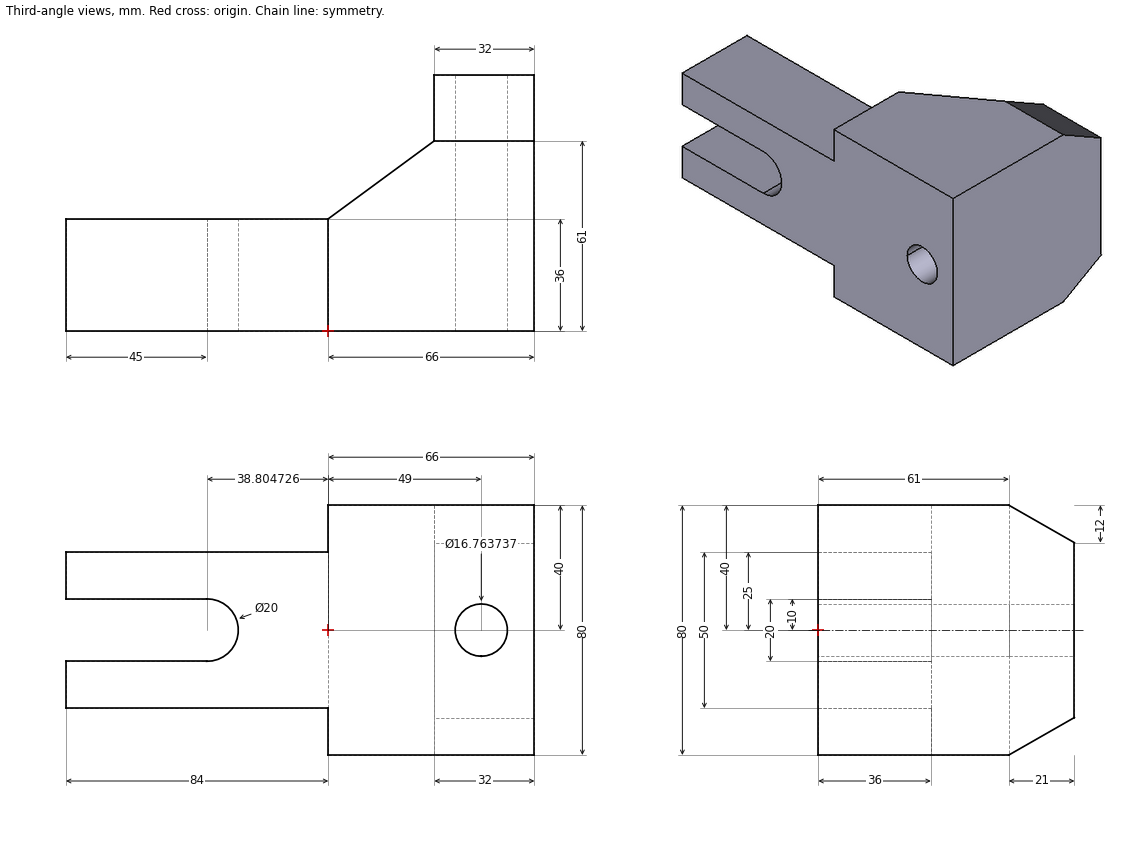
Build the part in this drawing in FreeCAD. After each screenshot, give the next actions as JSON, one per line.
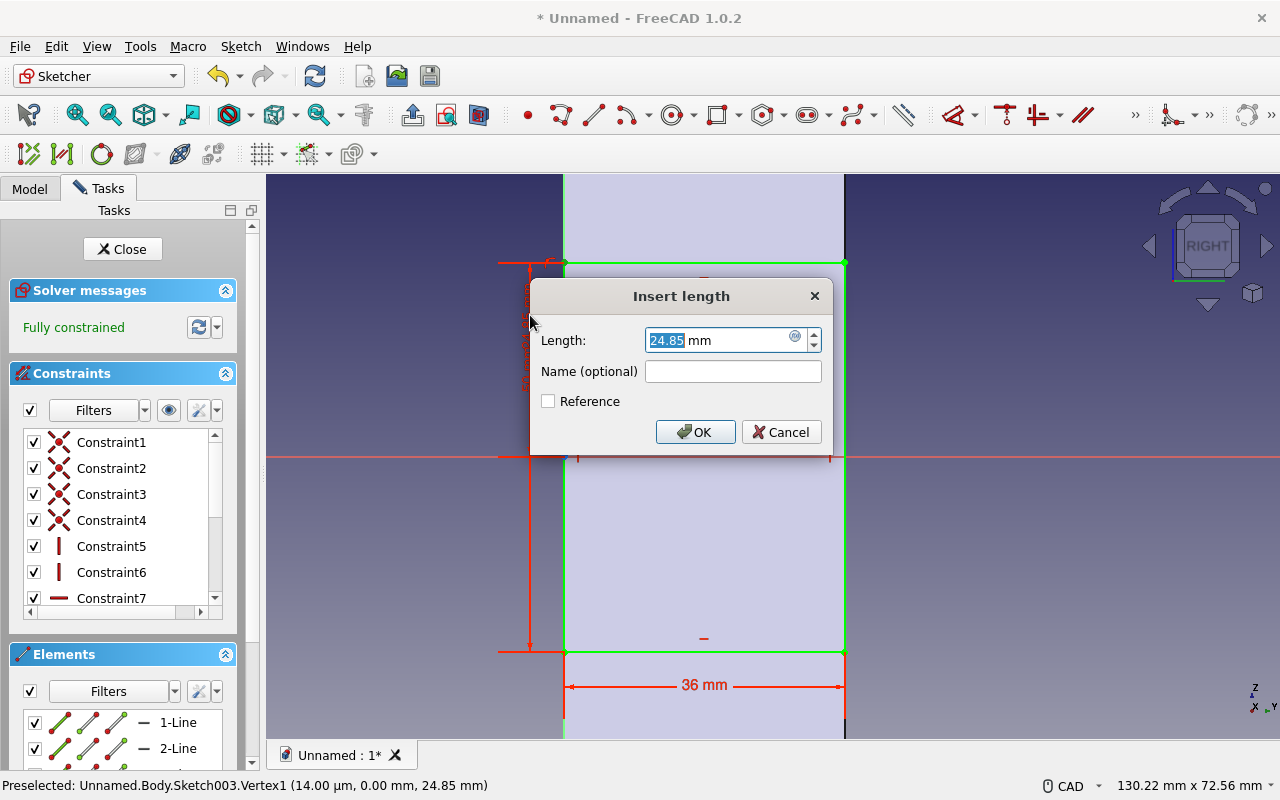
{"action": "type", "text": "25"}
{"action": "key", "text": "Return"}
{"action": "key", "text": "Escape"}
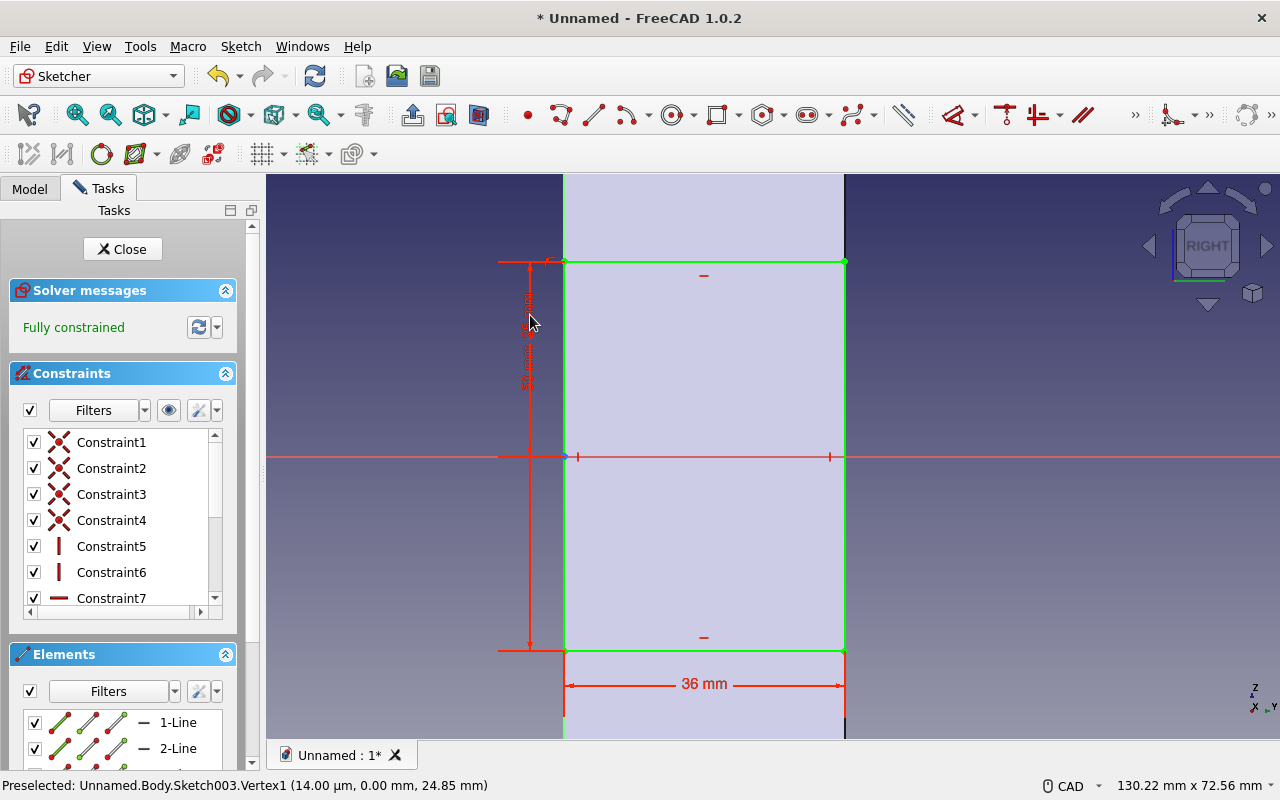
{"action": "left_click", "coordinate": [123, 249]}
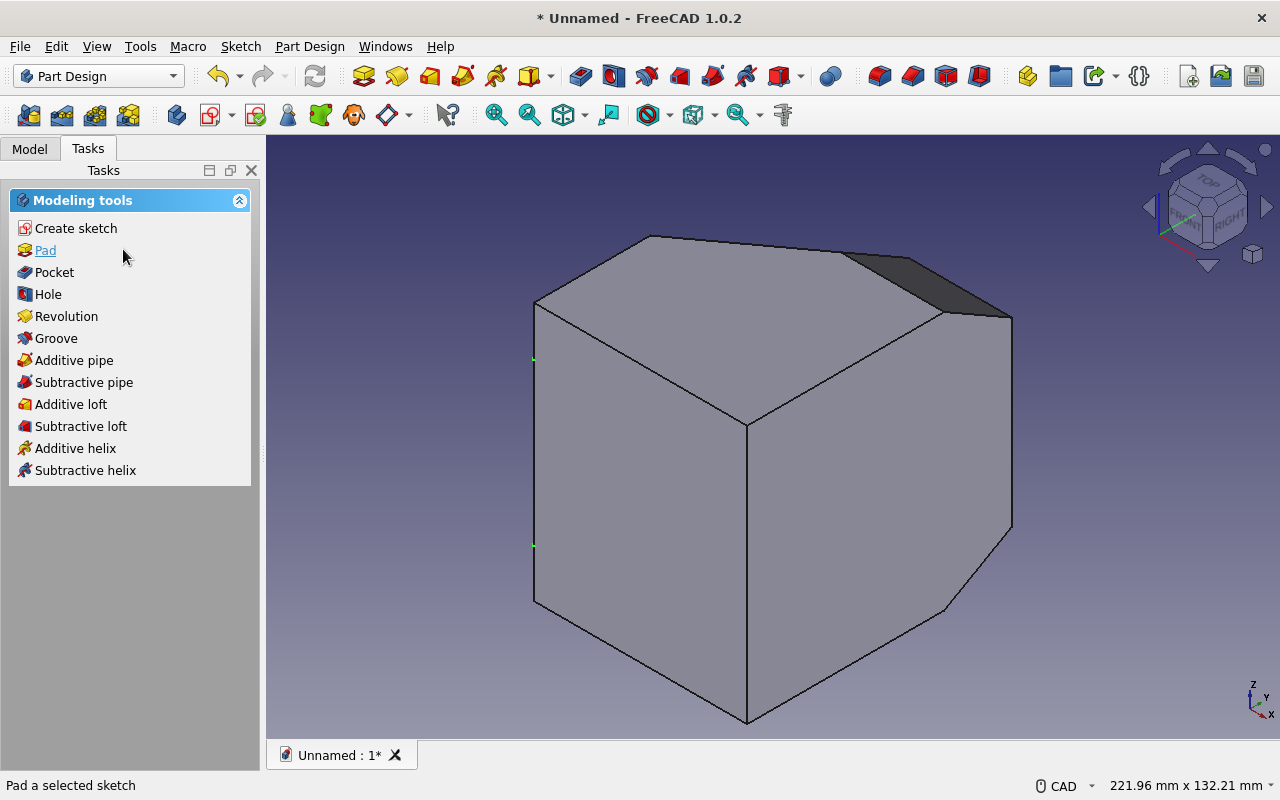
{"action": "left_click", "coordinate": [364, 76]}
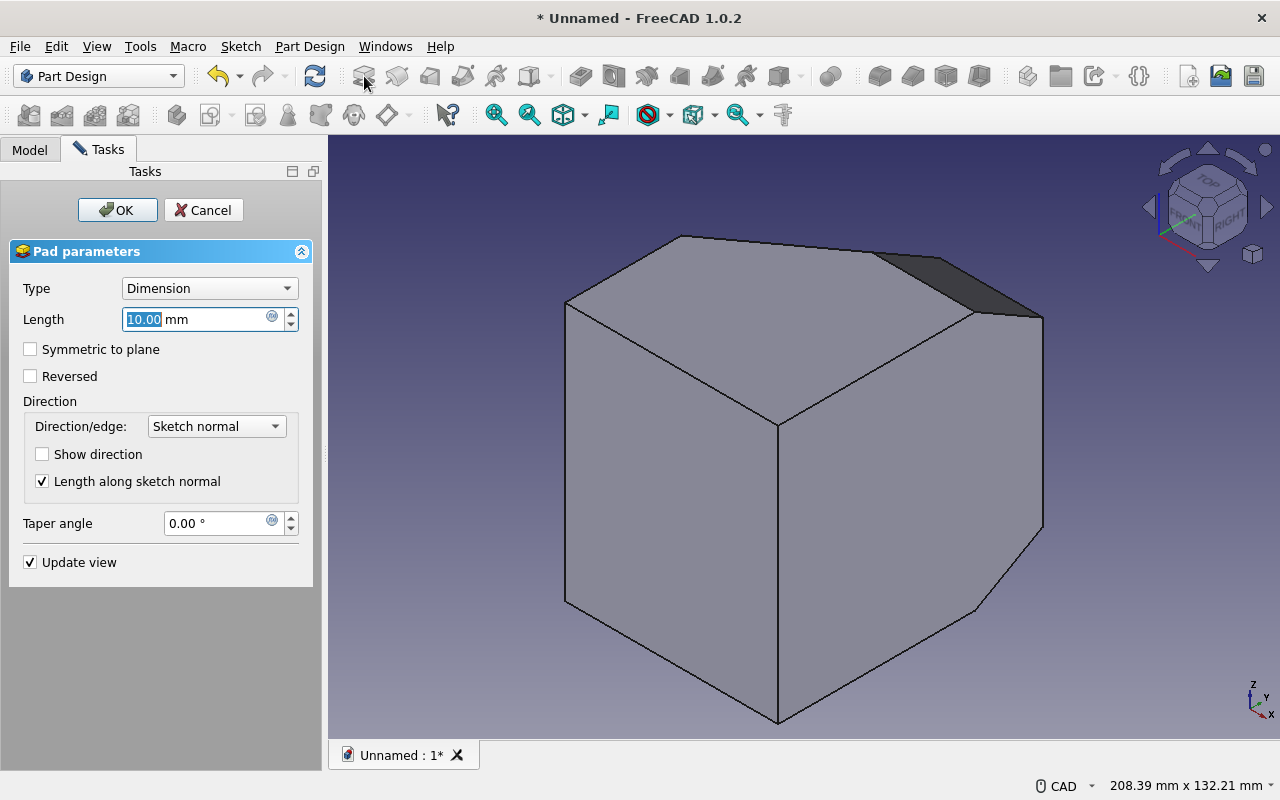
{"action": "type", "text": "84"}
{"action": "key", "text": "Tab"}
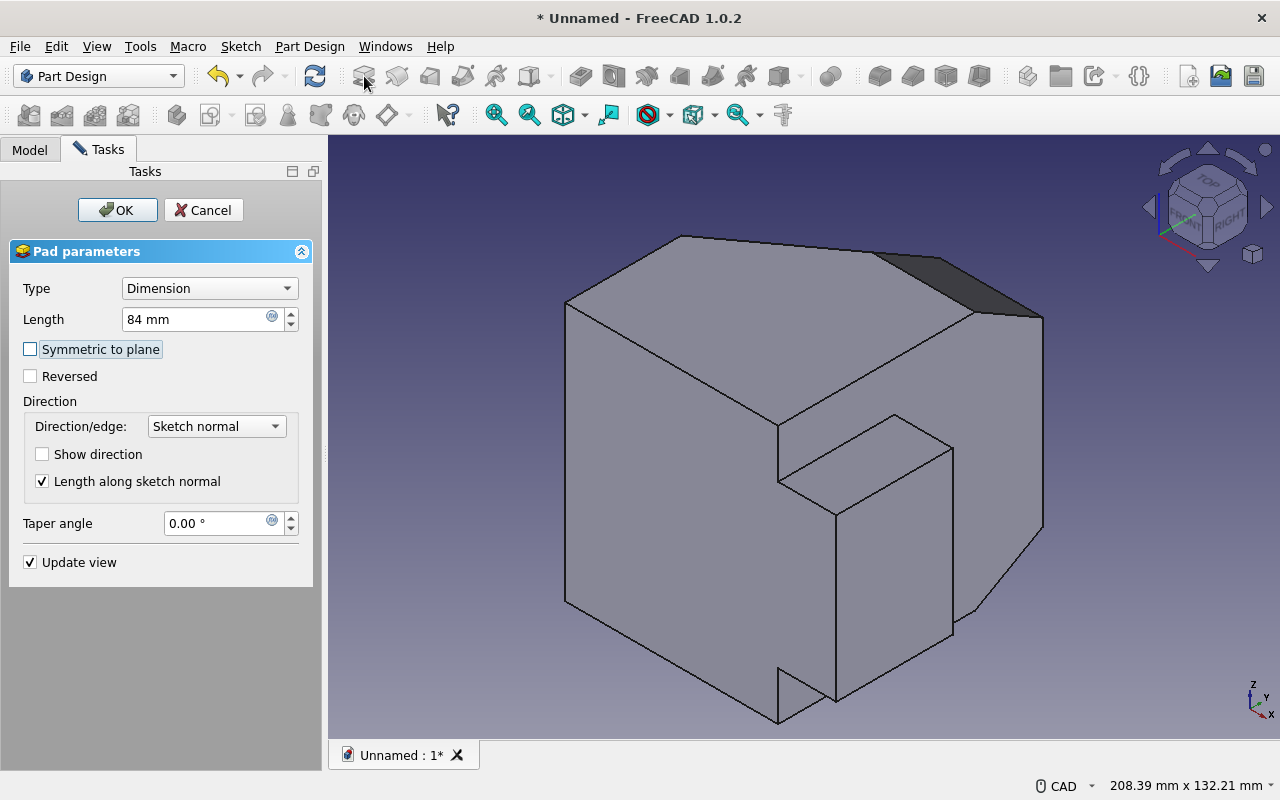
{"action": "left_click", "coordinate": [31, 376]}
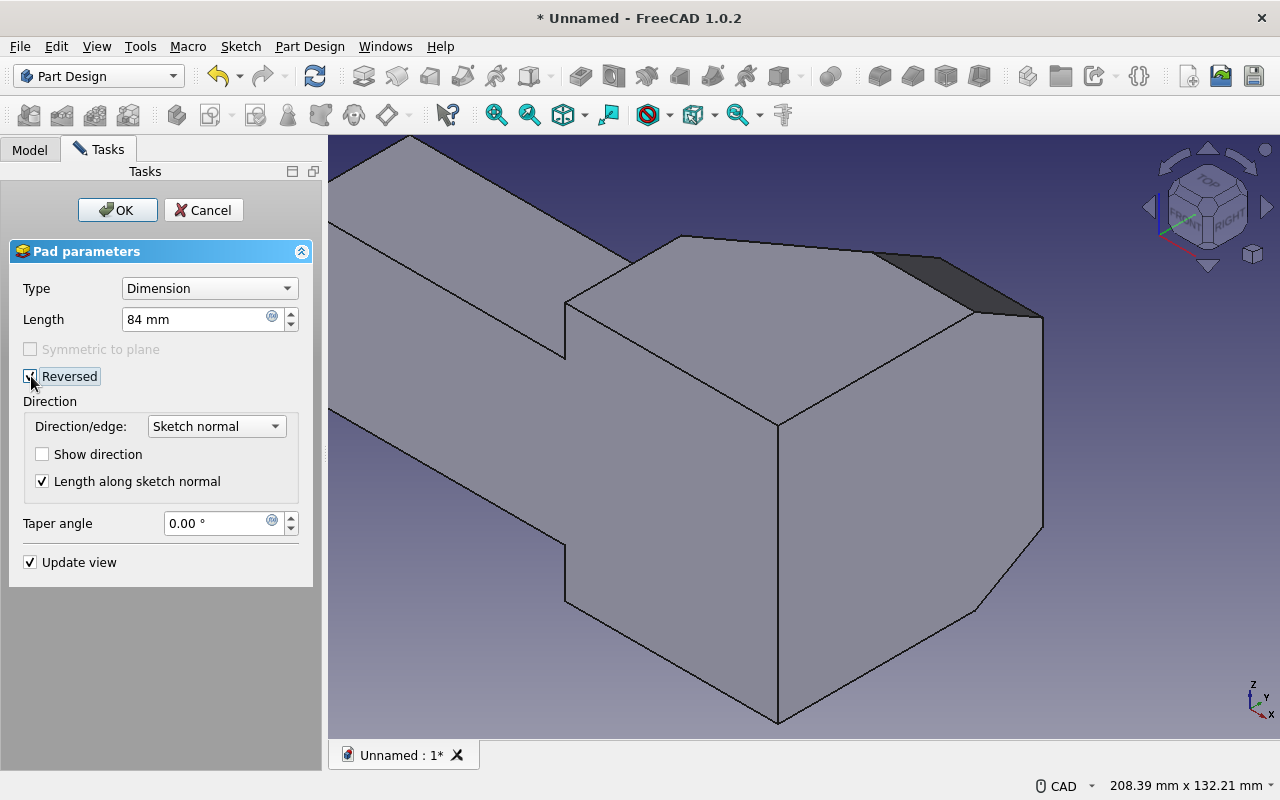
{"action": "left_click", "coordinate": [118, 210]}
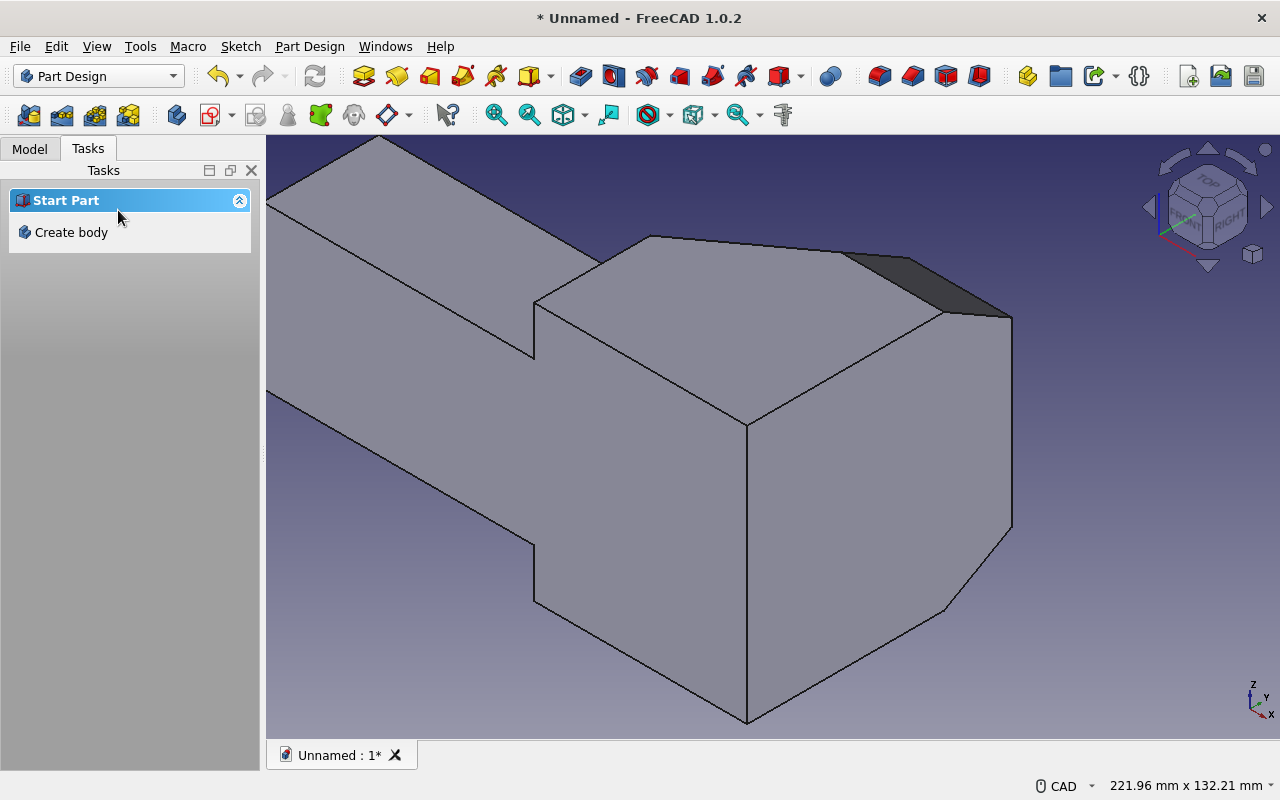
{"action": "left_click", "coordinate": [497, 116]}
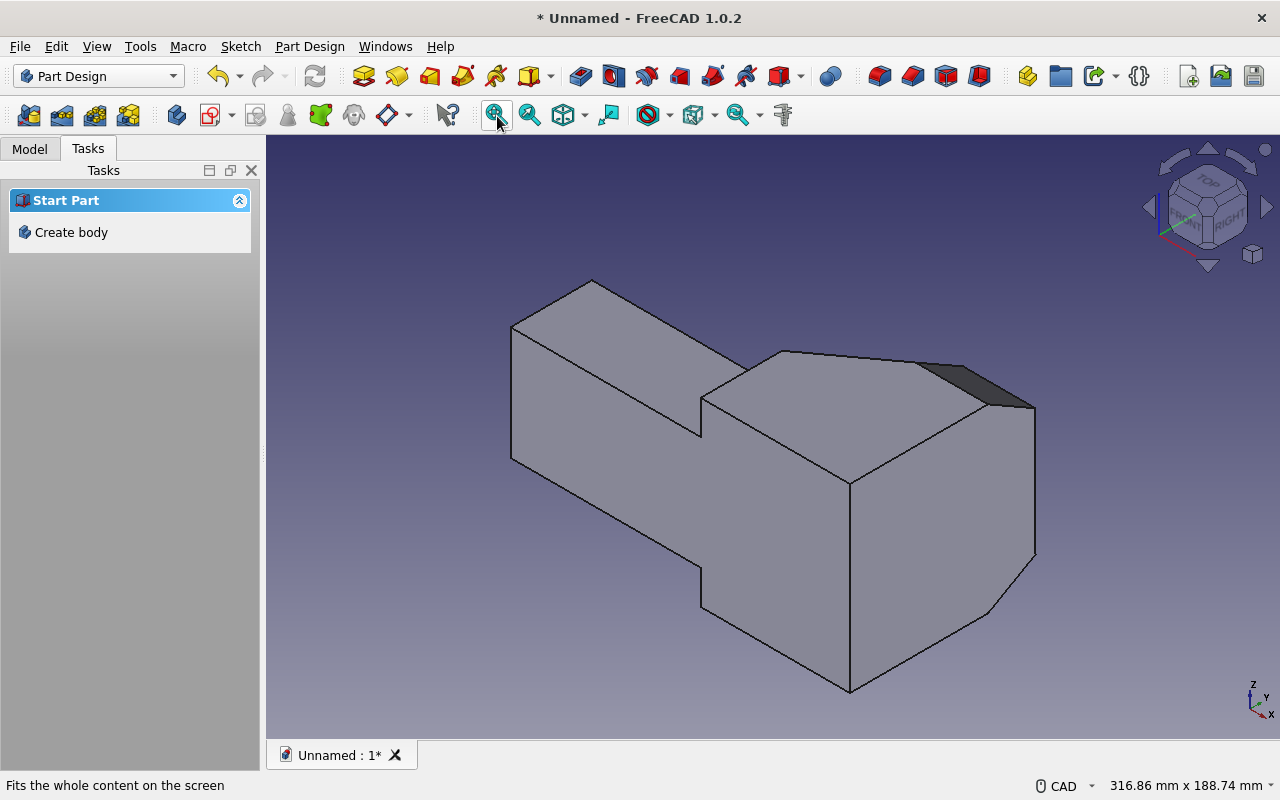
{"action": "key", "text": "6"}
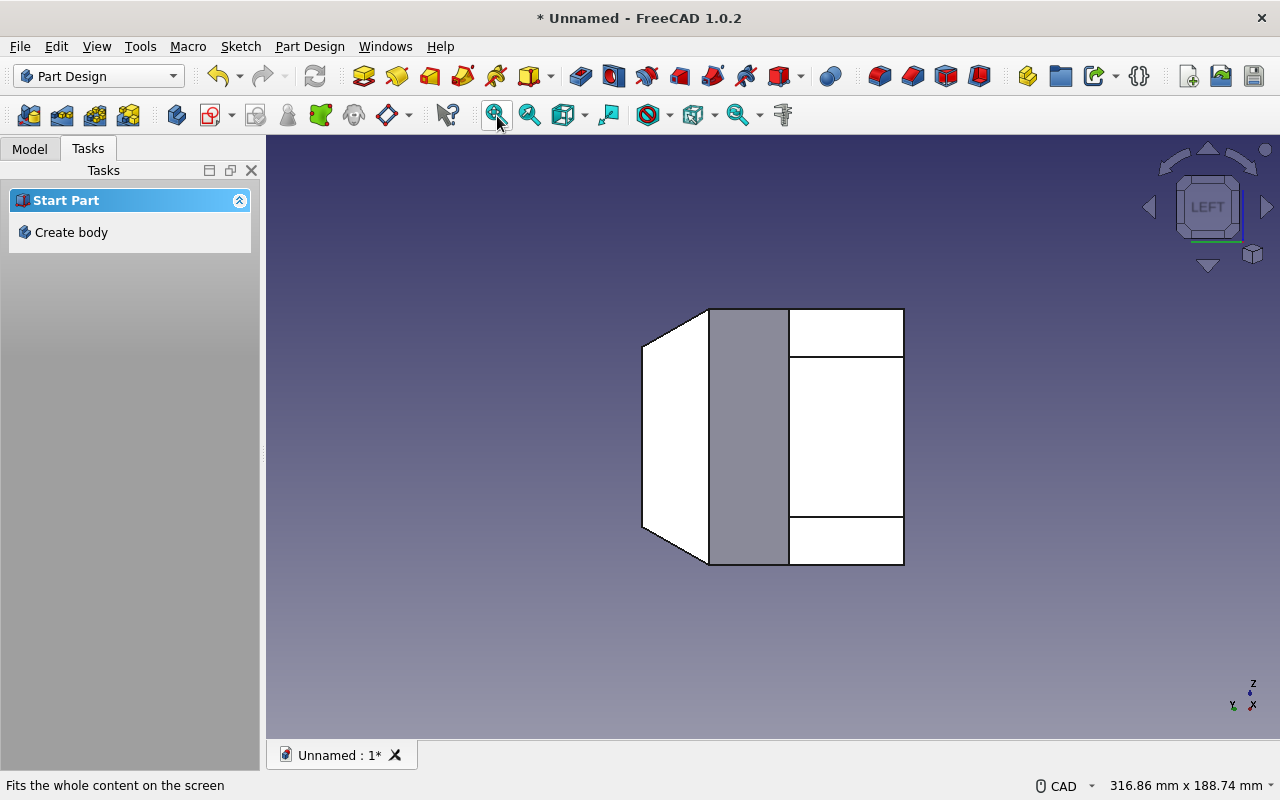
{"action": "left_click", "coordinate": [497, 116]}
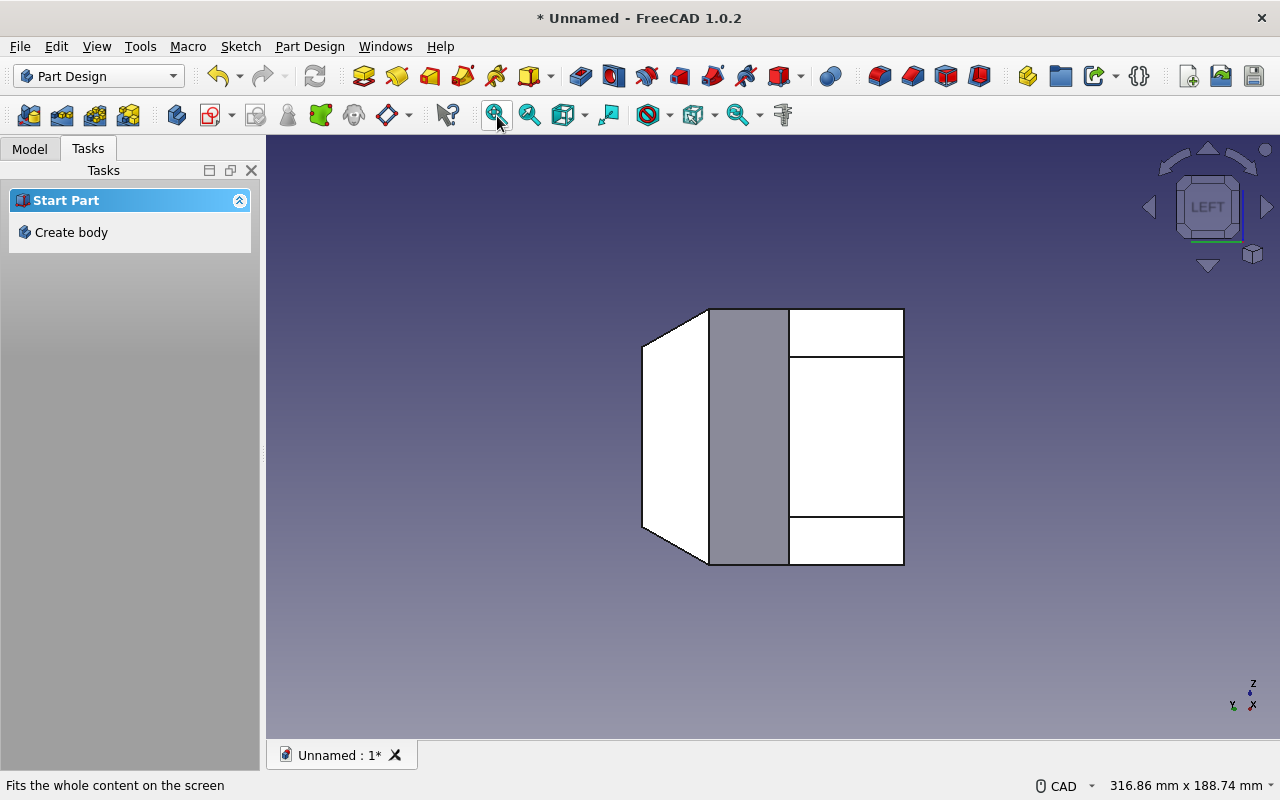
{"action": "left_click", "coordinate": [847, 436]}